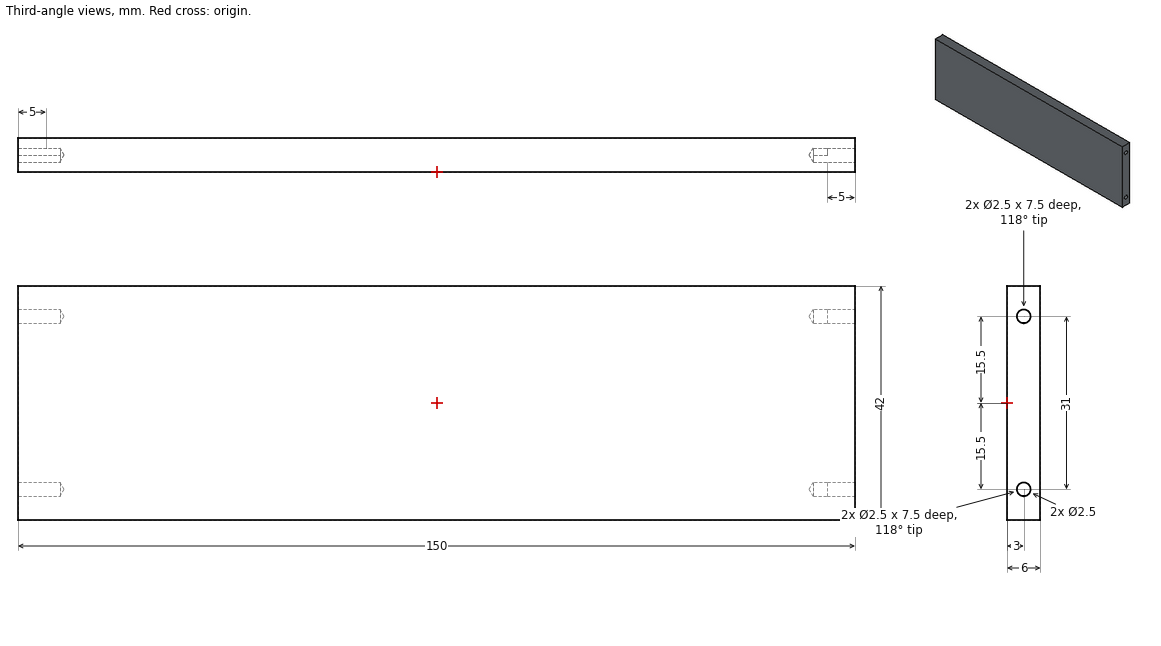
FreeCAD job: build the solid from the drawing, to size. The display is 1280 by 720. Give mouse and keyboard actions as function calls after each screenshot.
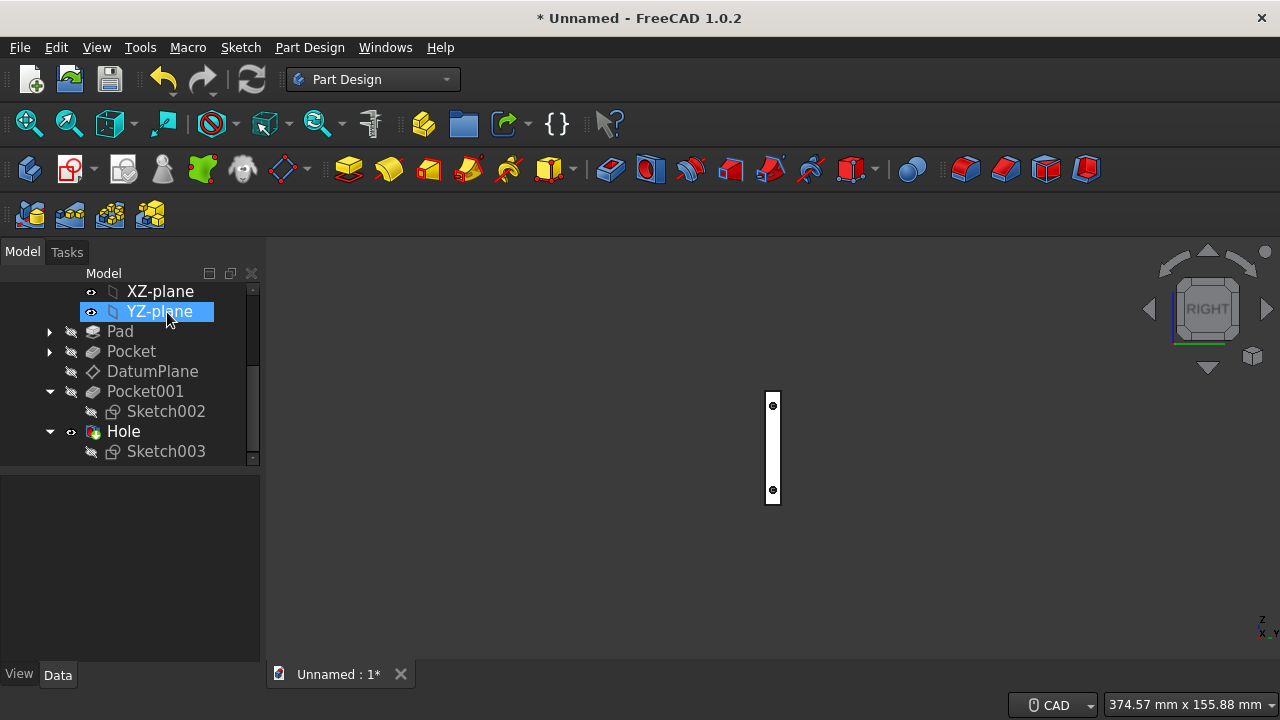
key(6)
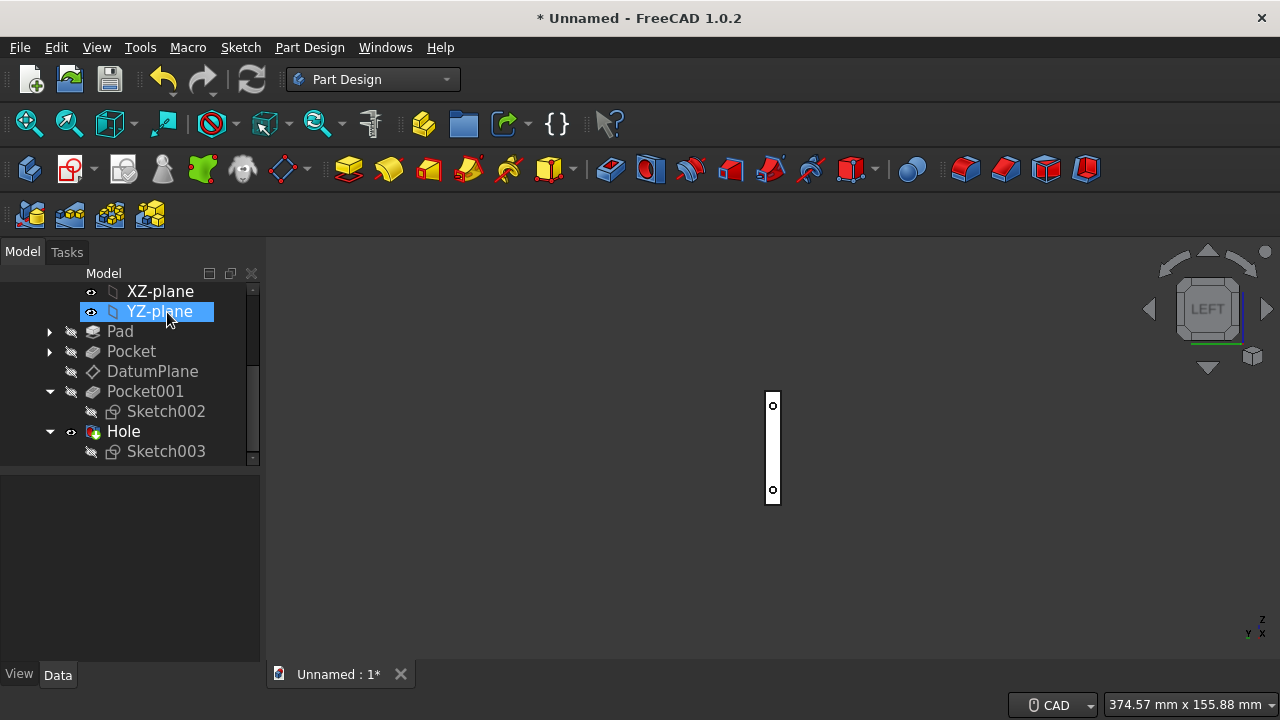
click(30, 124)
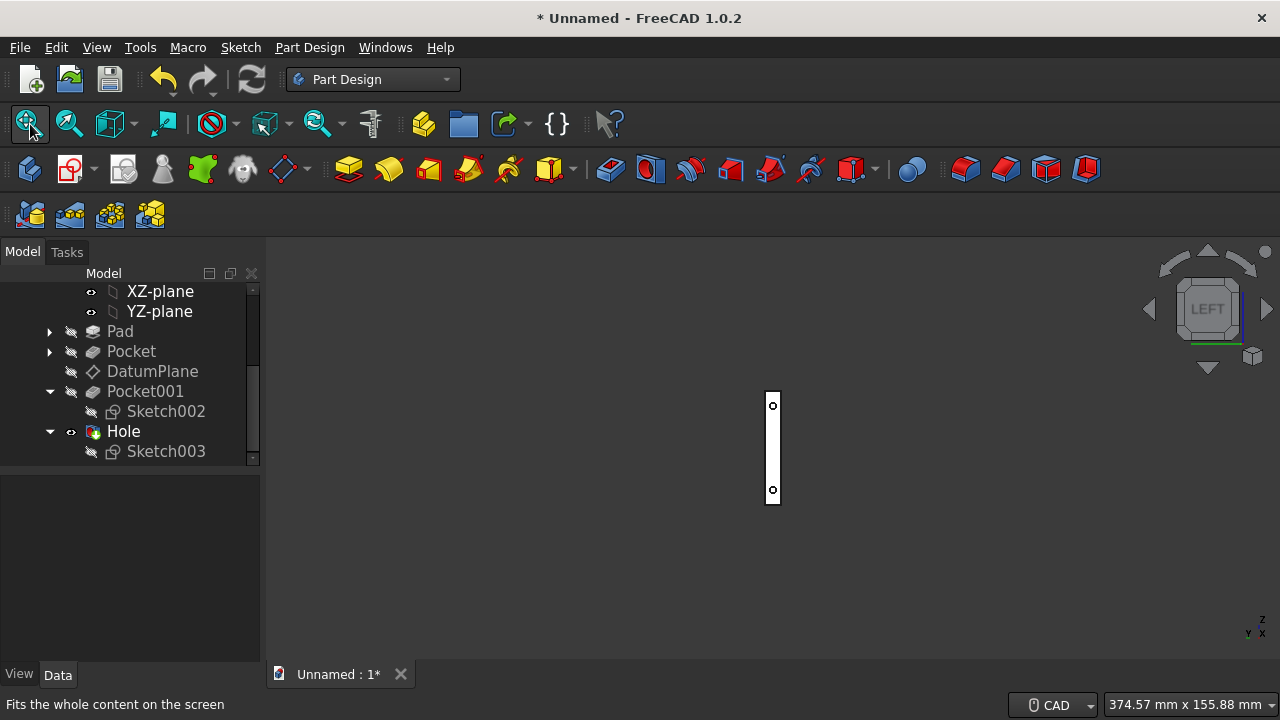
click(773, 447)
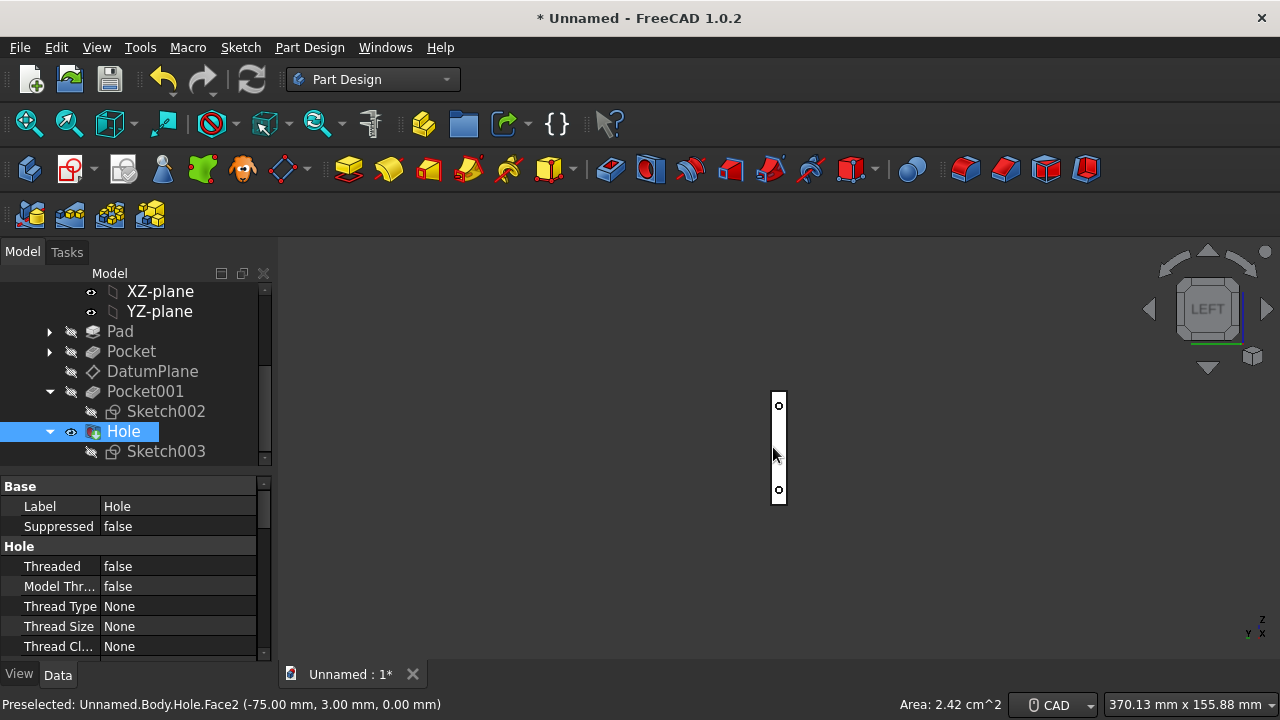
click(70, 170)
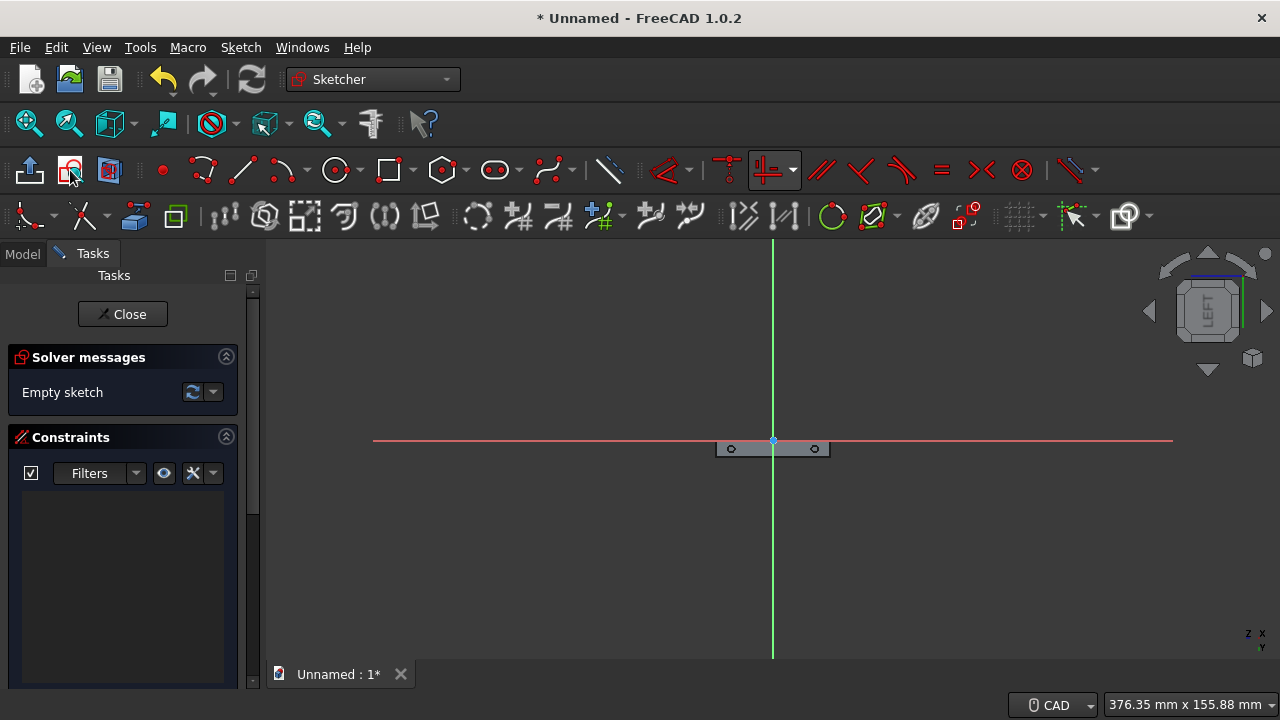
scroll(787, 446, up, 9)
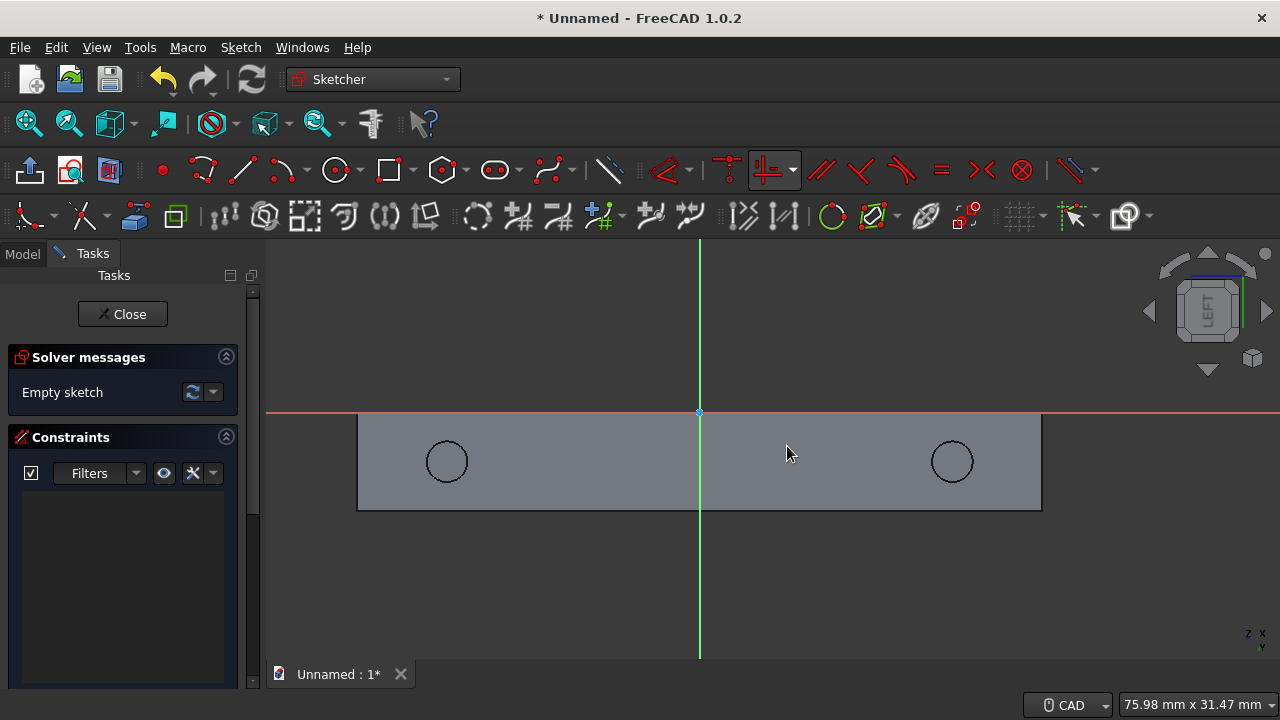
click(336, 170)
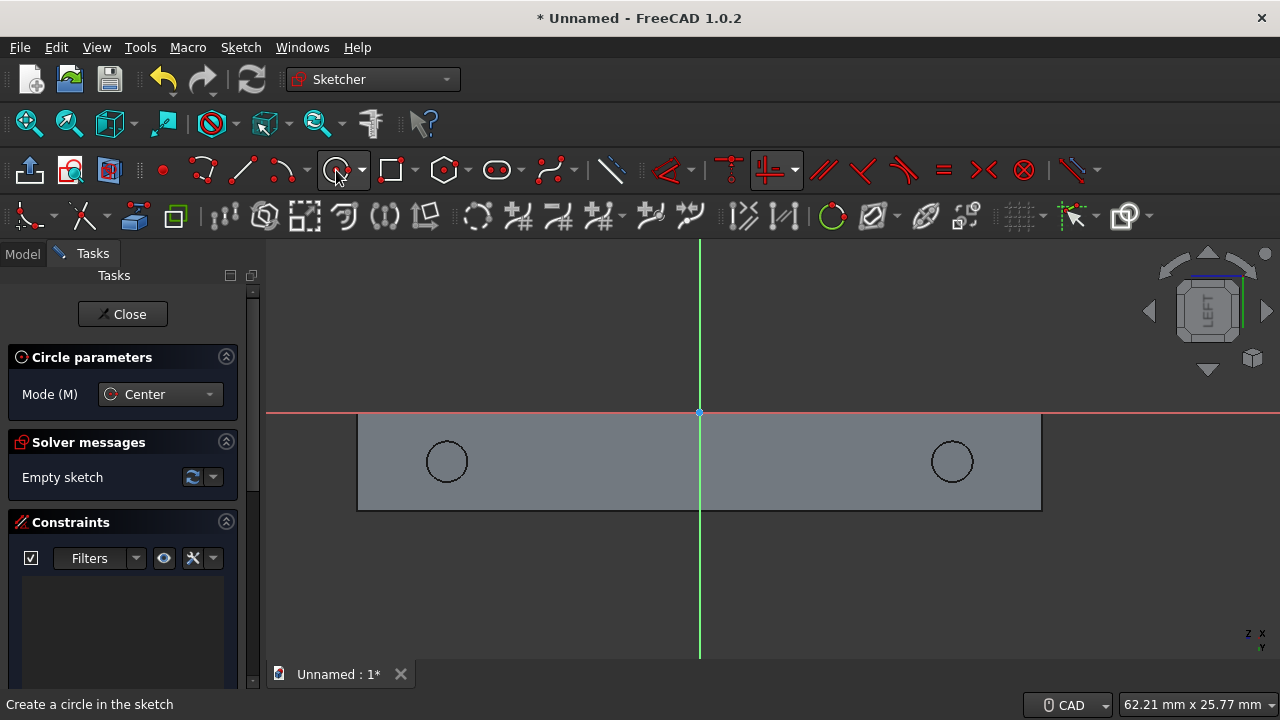
click(952, 462)
move(967, 447)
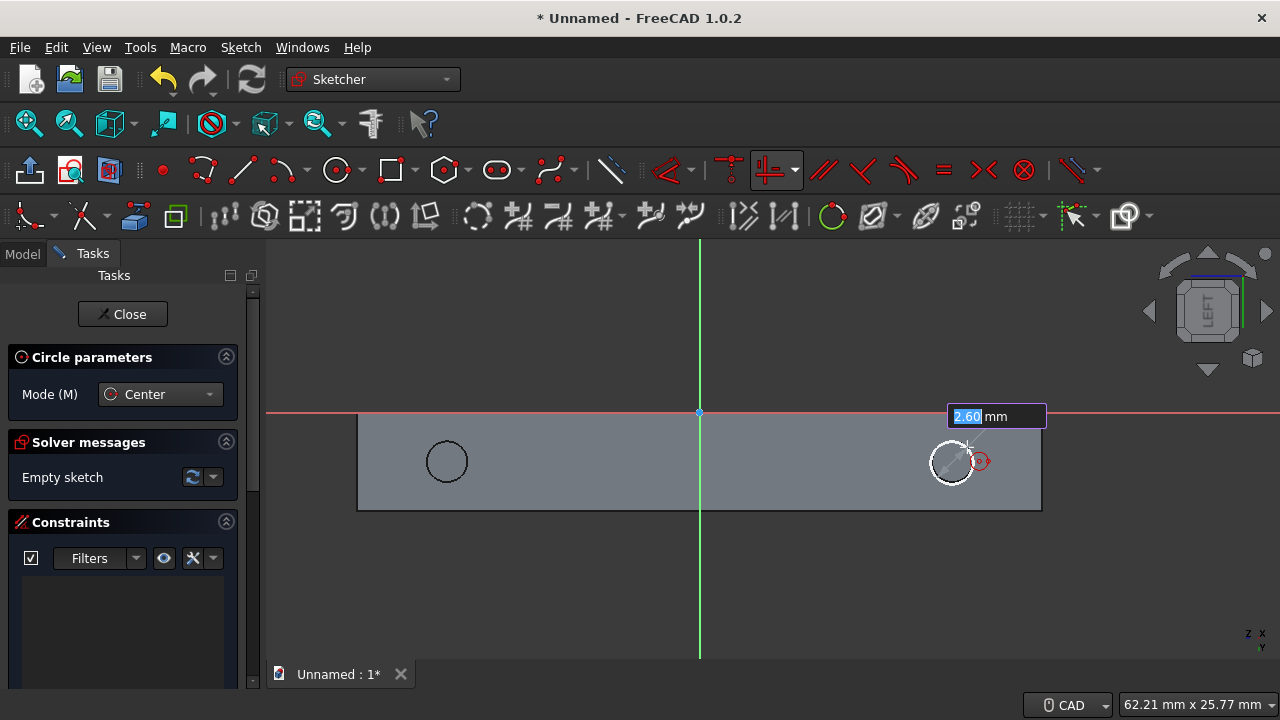
text(2.5)
key(Return)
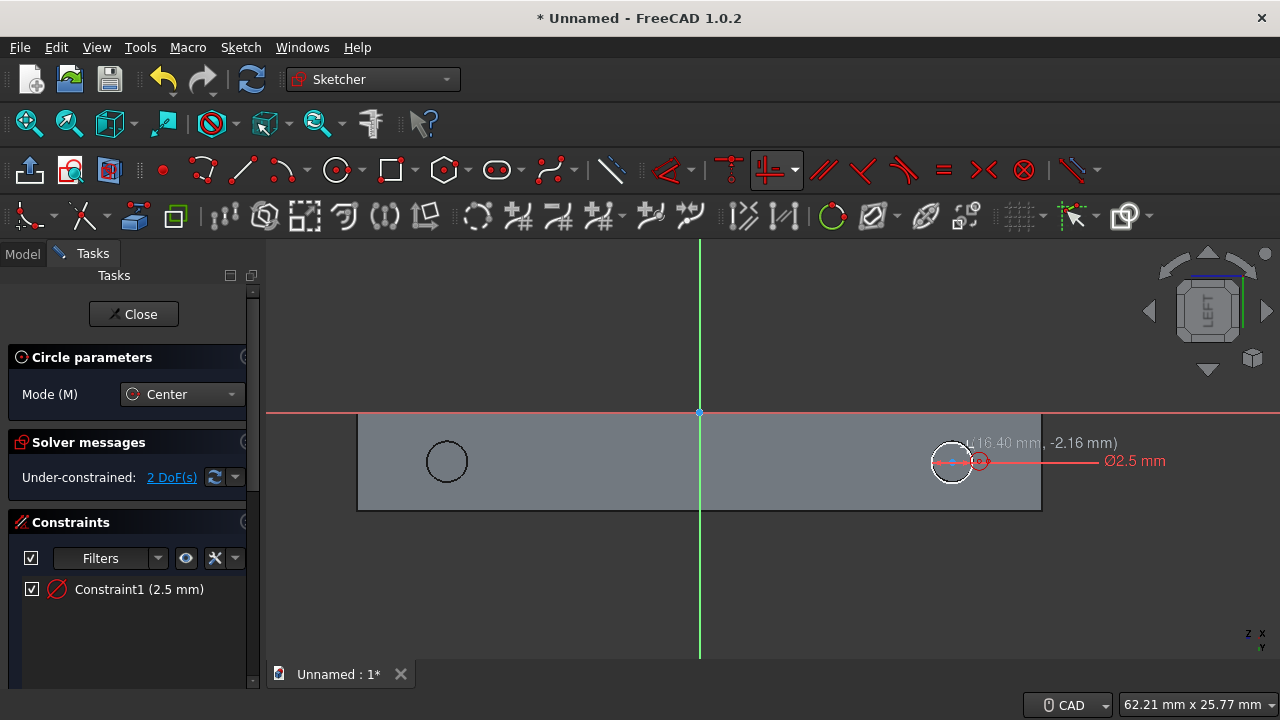
click(447, 462)
move(461, 447)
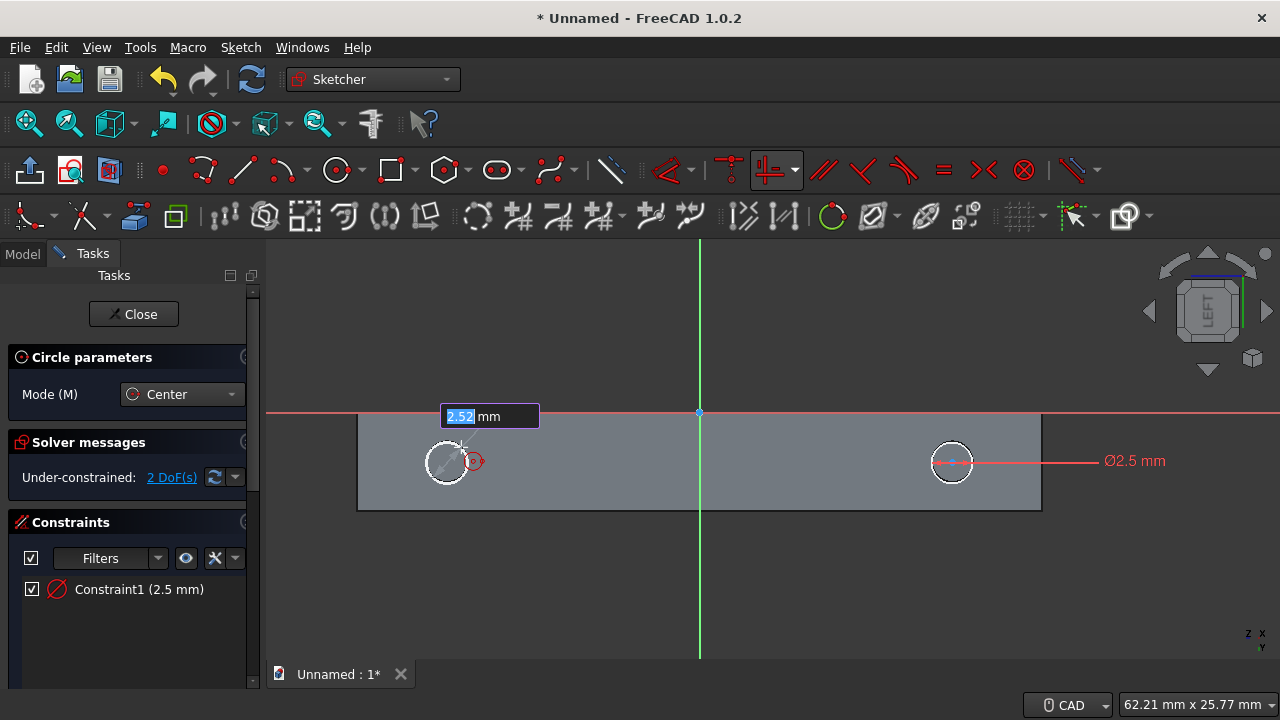
text(2.5)
key(Return)
key(Escape)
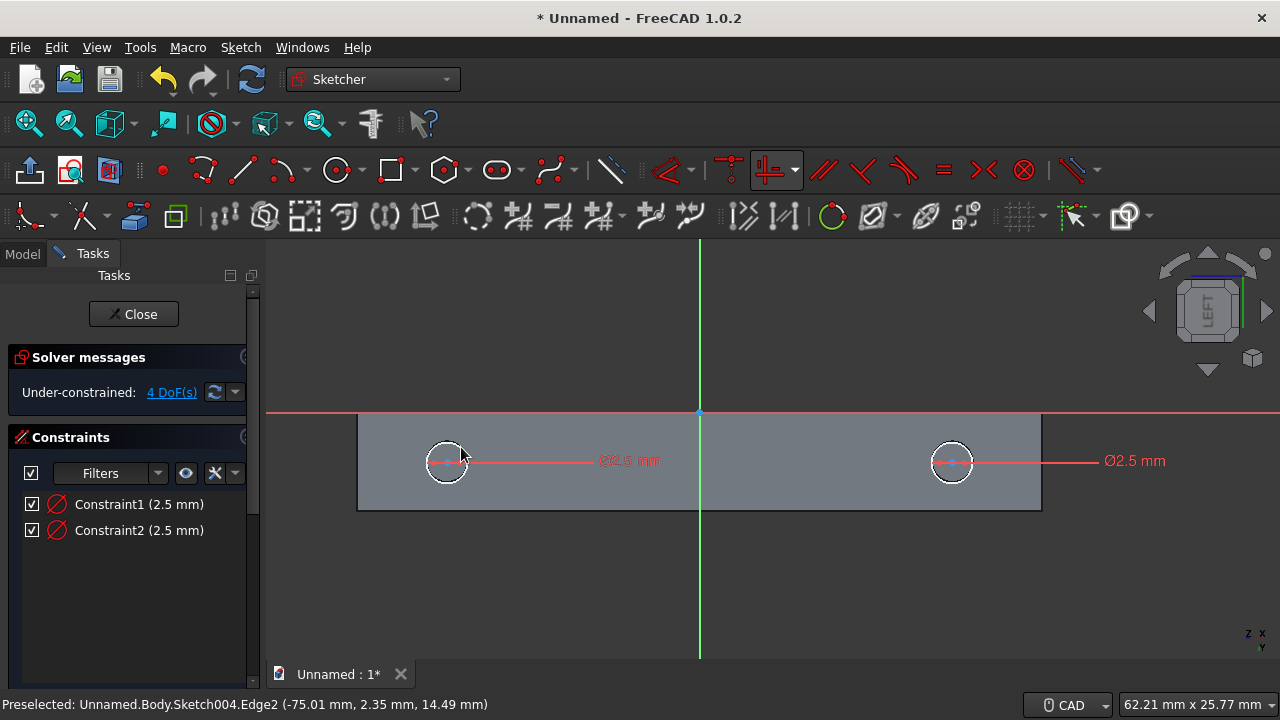
click(952, 463)